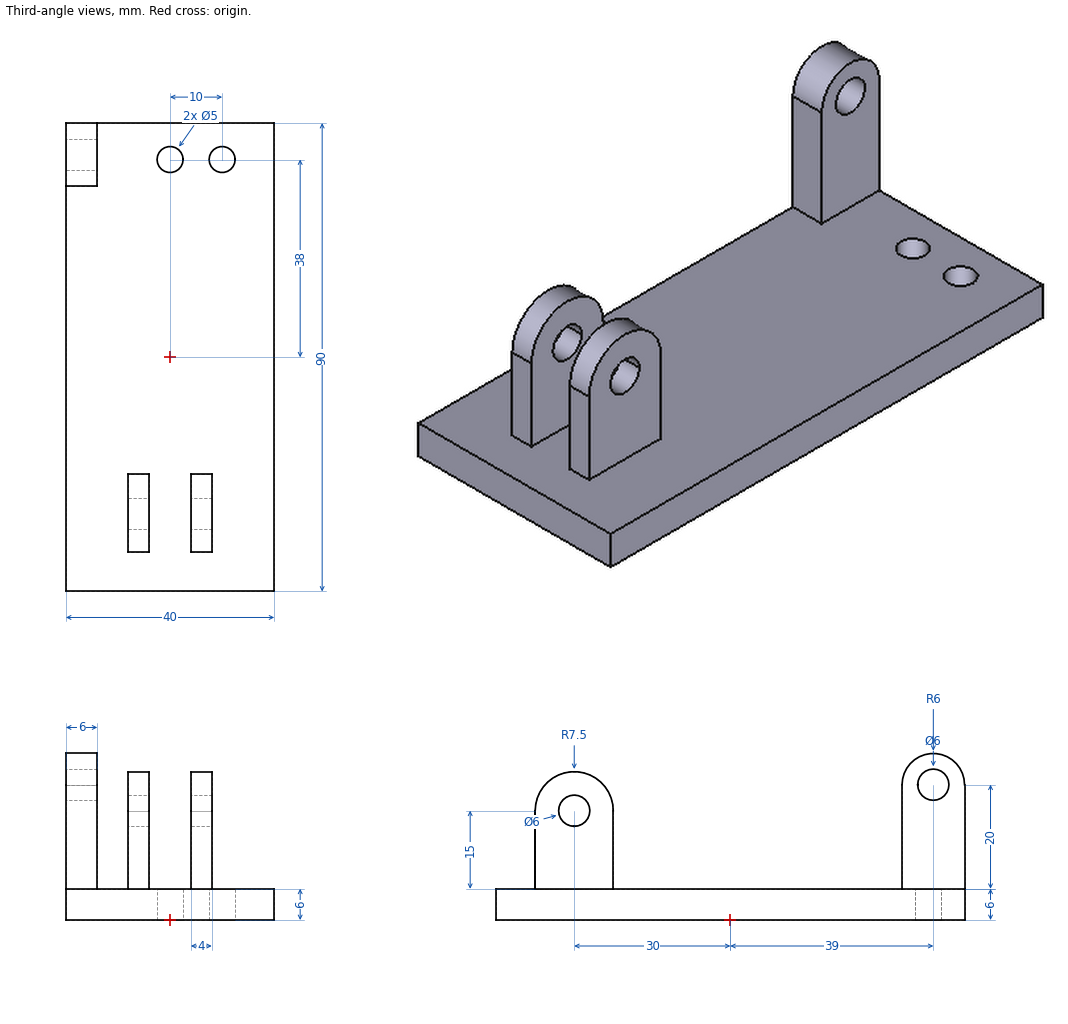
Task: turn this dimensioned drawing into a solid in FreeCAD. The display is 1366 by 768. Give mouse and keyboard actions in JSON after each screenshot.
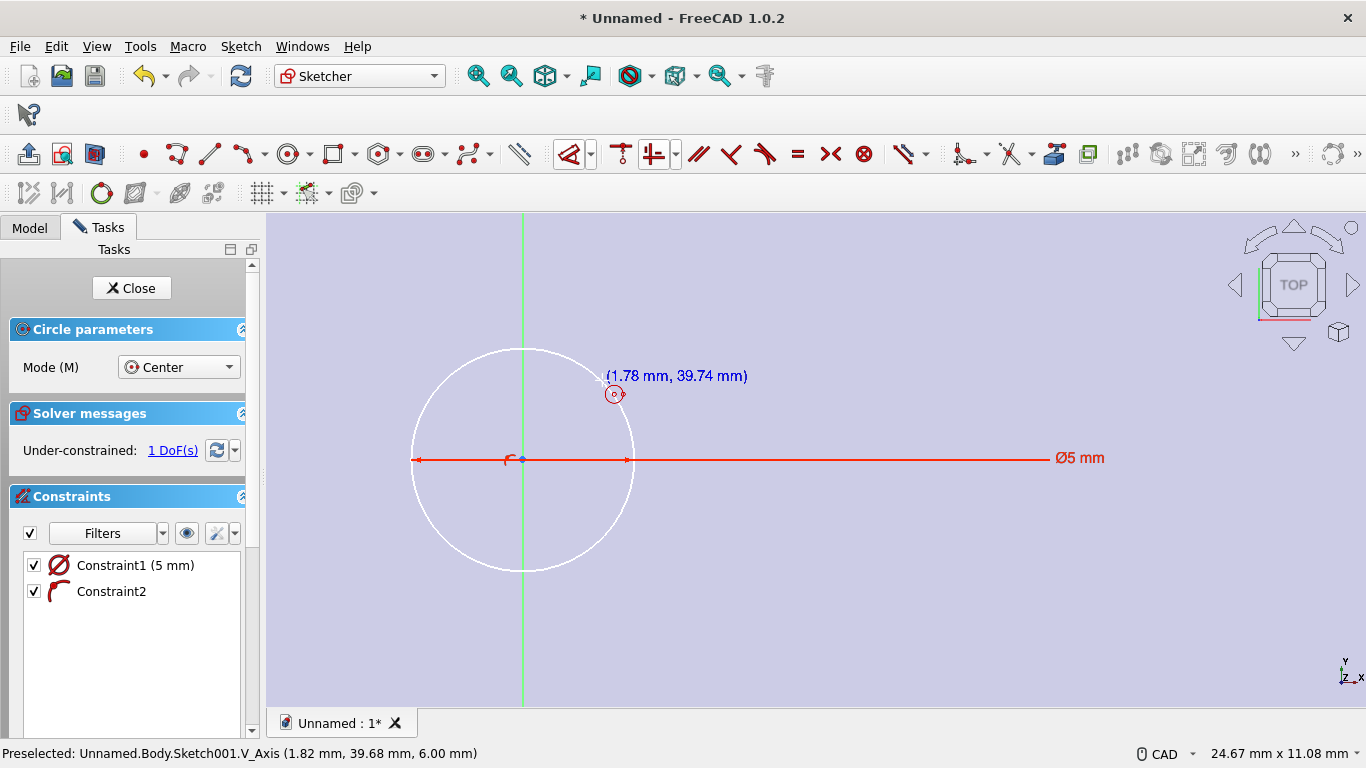
{"action": "left_click", "coordinate": [969, 459]}
{"action": "mouse_move", "coordinate": [1047, 380]}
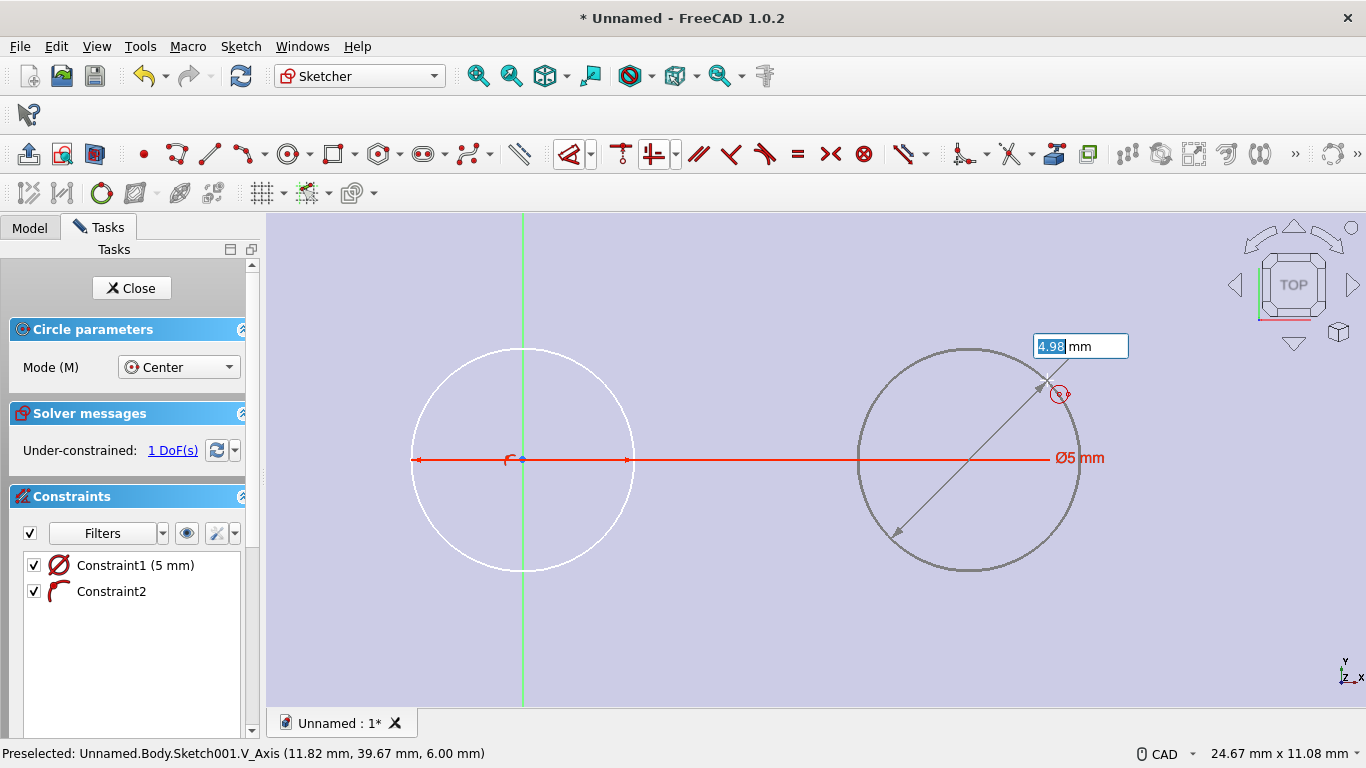
{"action": "type", "text": "5"}
{"action": "key", "text": "Return"}
{"action": "key", "text": "Escape"}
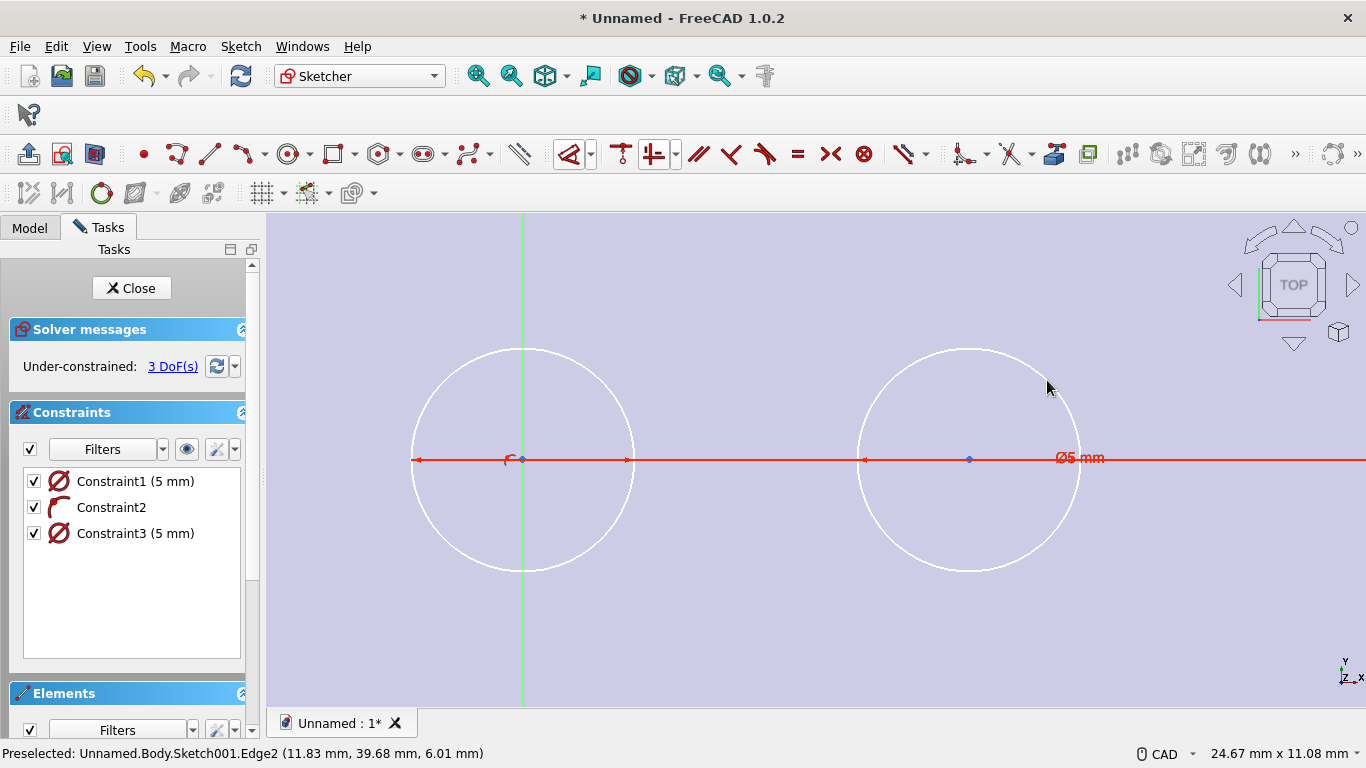
{"action": "left_click", "coordinate": [523, 460]}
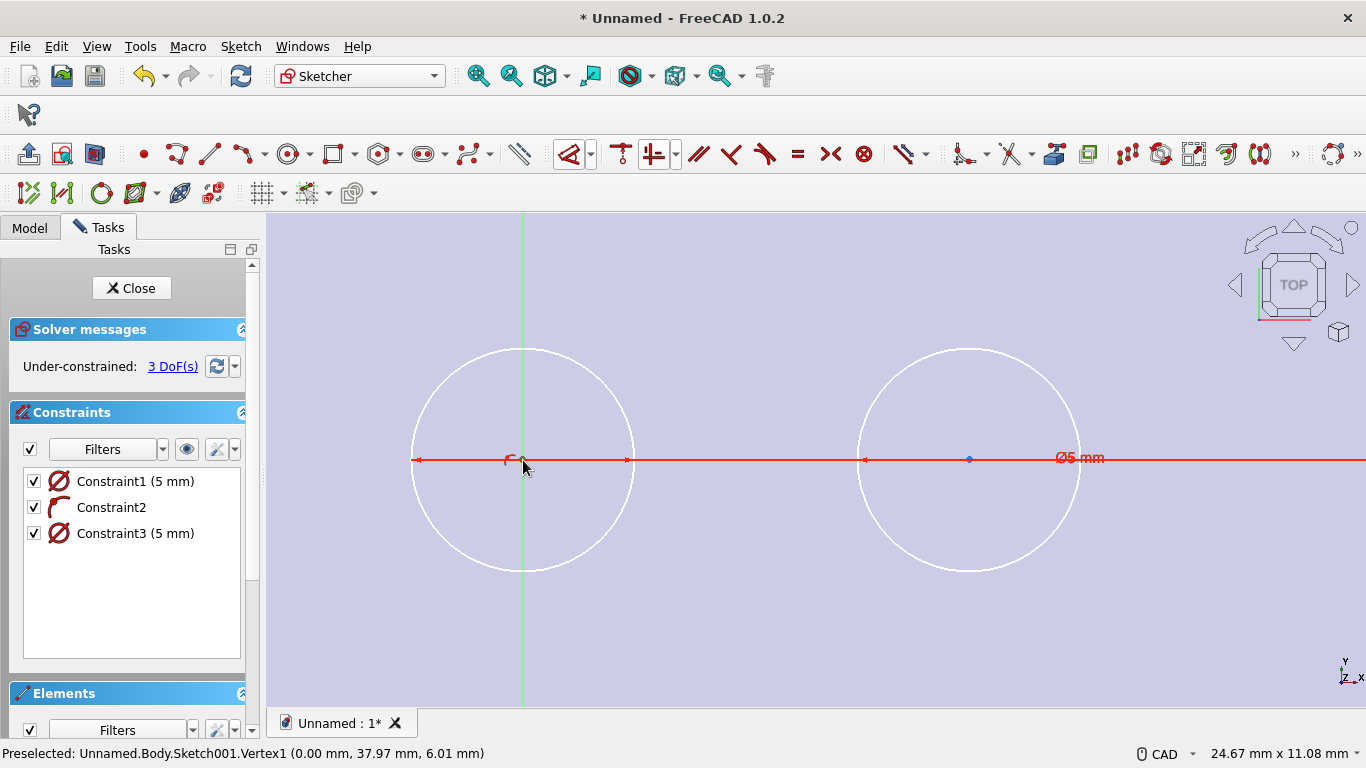
{"action": "left_click", "coordinate": [969, 460]}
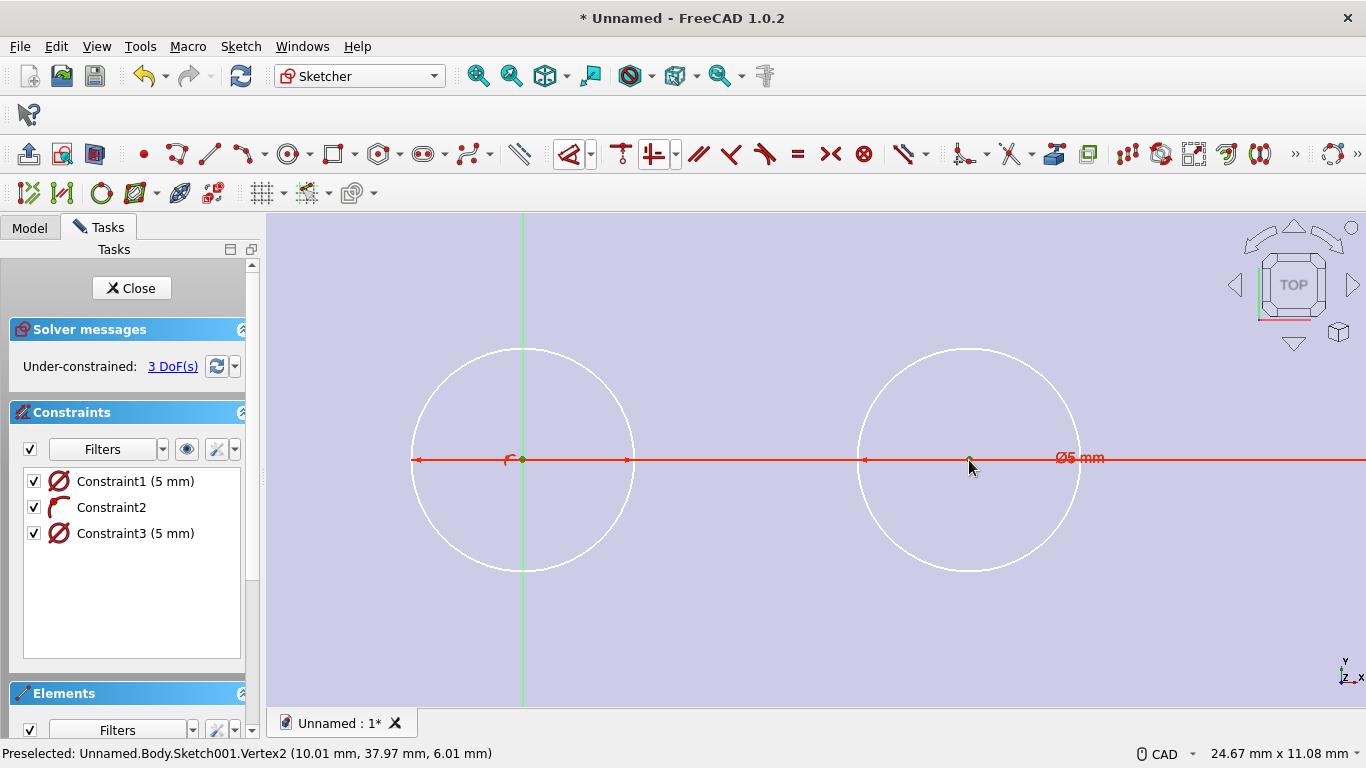
{"action": "key", "text": "h"}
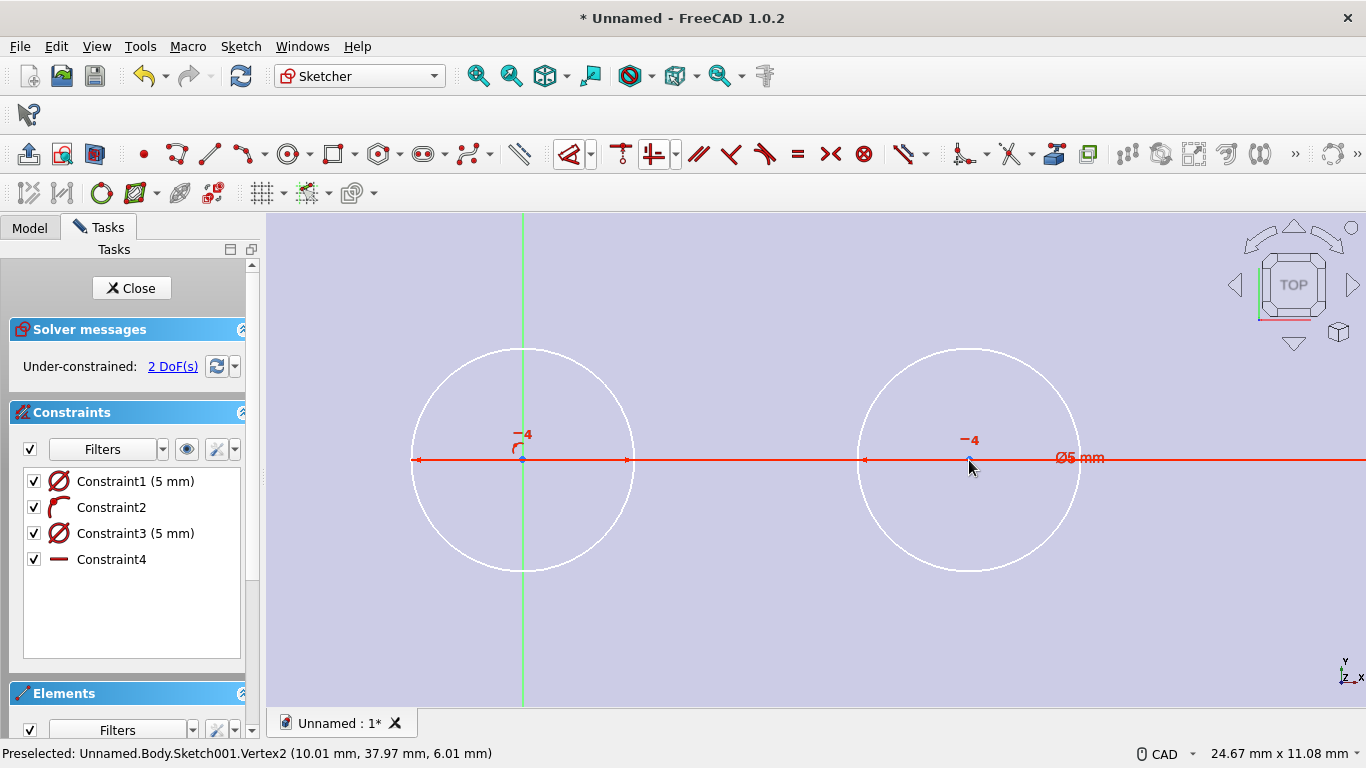
{"action": "key", "text": "d"}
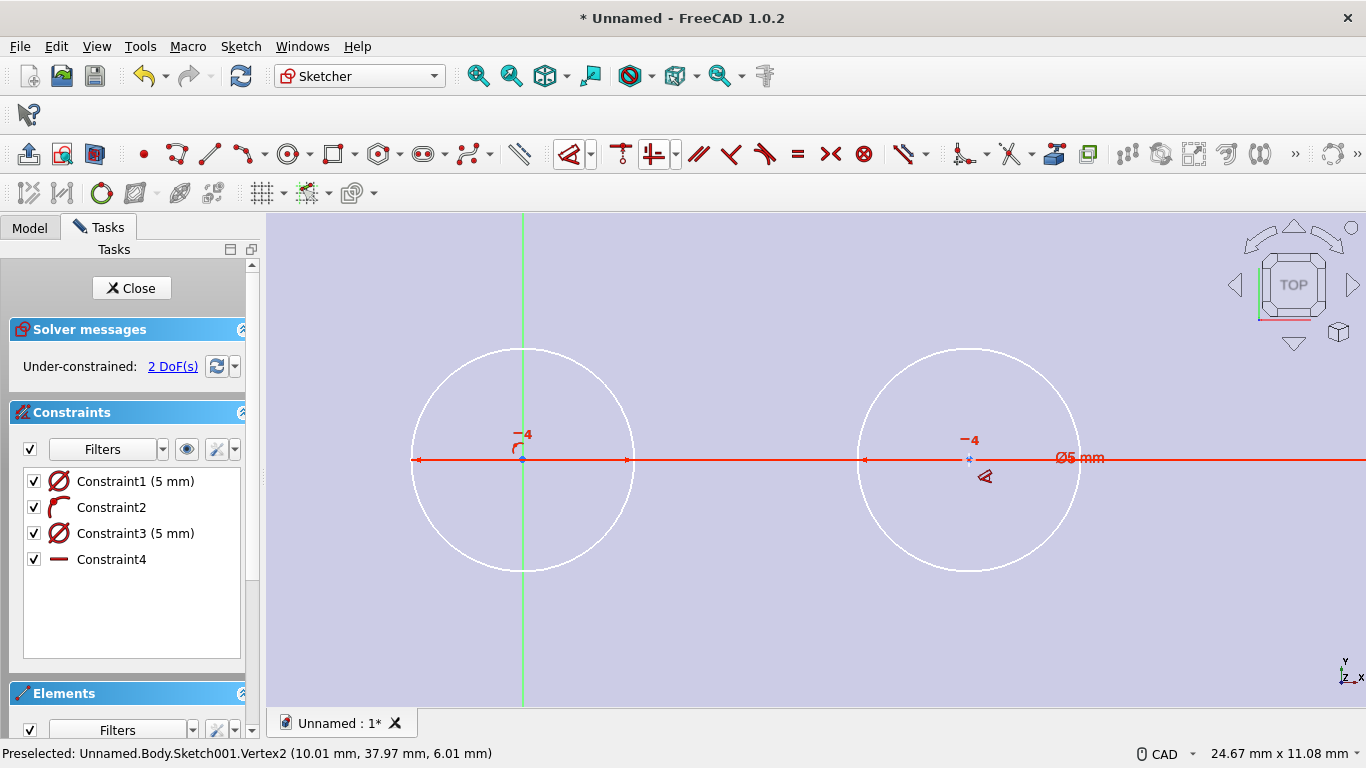
{"action": "left_click", "coordinate": [523, 460]}
{"action": "left_click", "coordinate": [489, 519]}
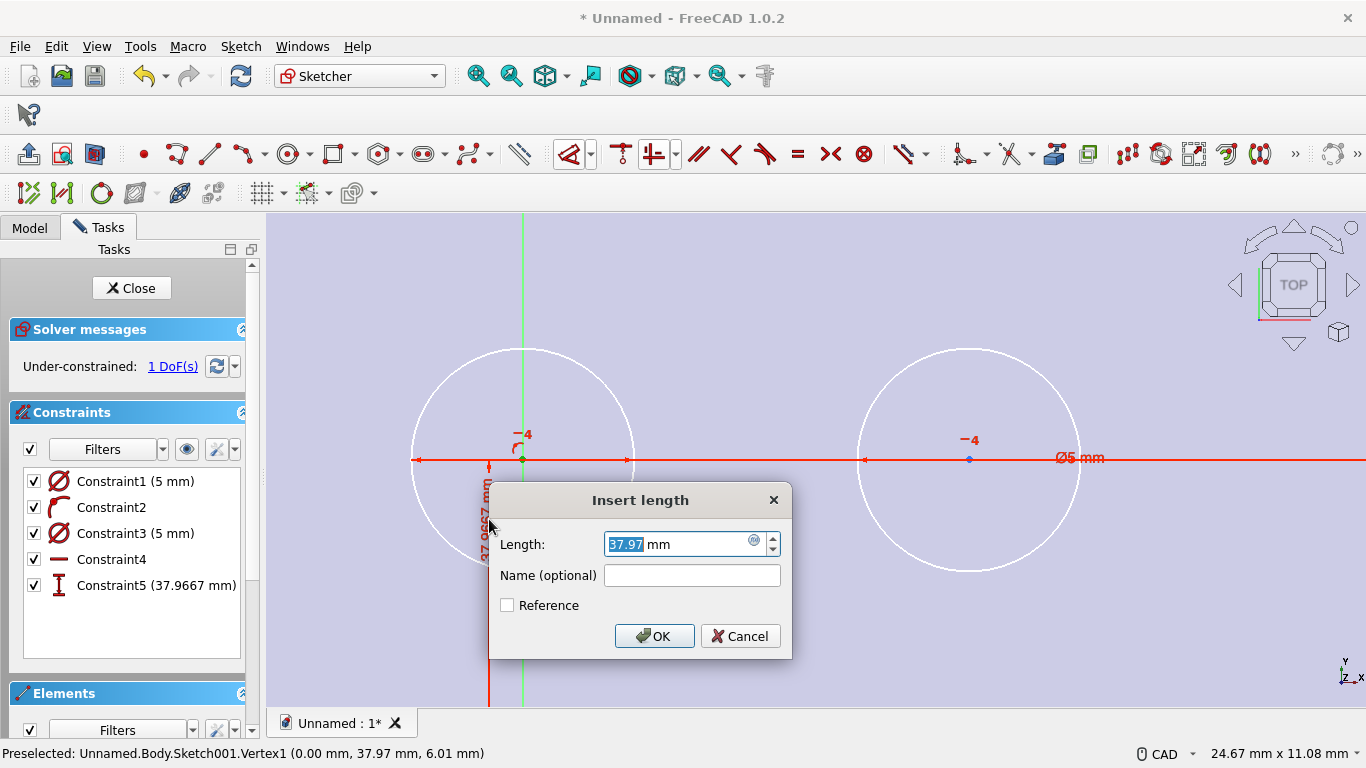
{"action": "type", "text": "38"}
{"action": "key", "text": "Return"}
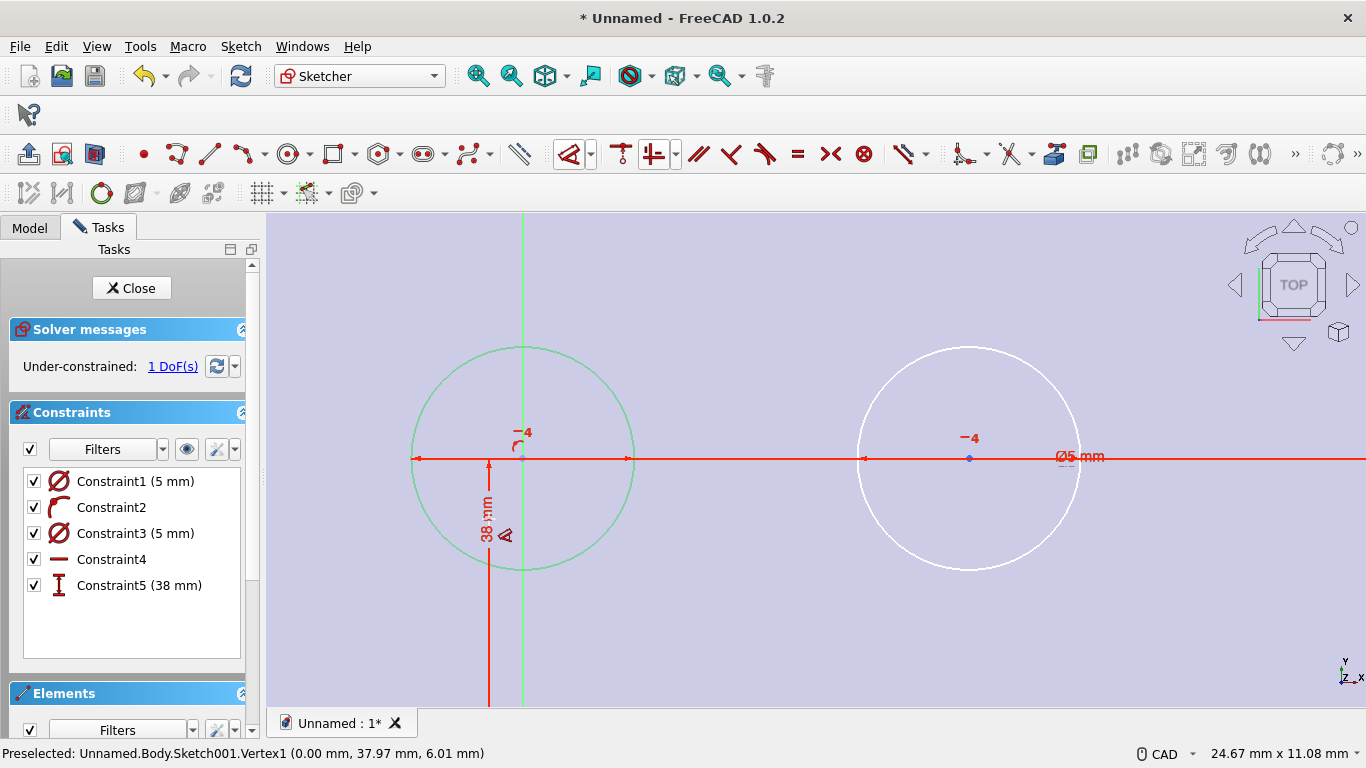
{"action": "left_click", "coordinate": [969, 459]}
{"action": "left_click", "coordinate": [746, 425]}